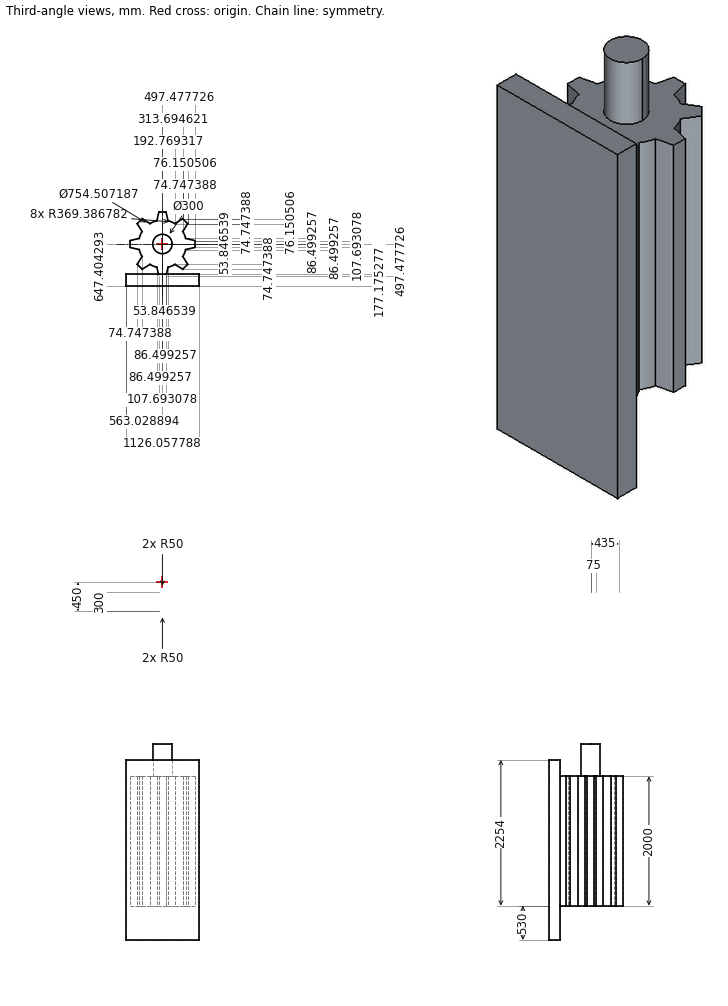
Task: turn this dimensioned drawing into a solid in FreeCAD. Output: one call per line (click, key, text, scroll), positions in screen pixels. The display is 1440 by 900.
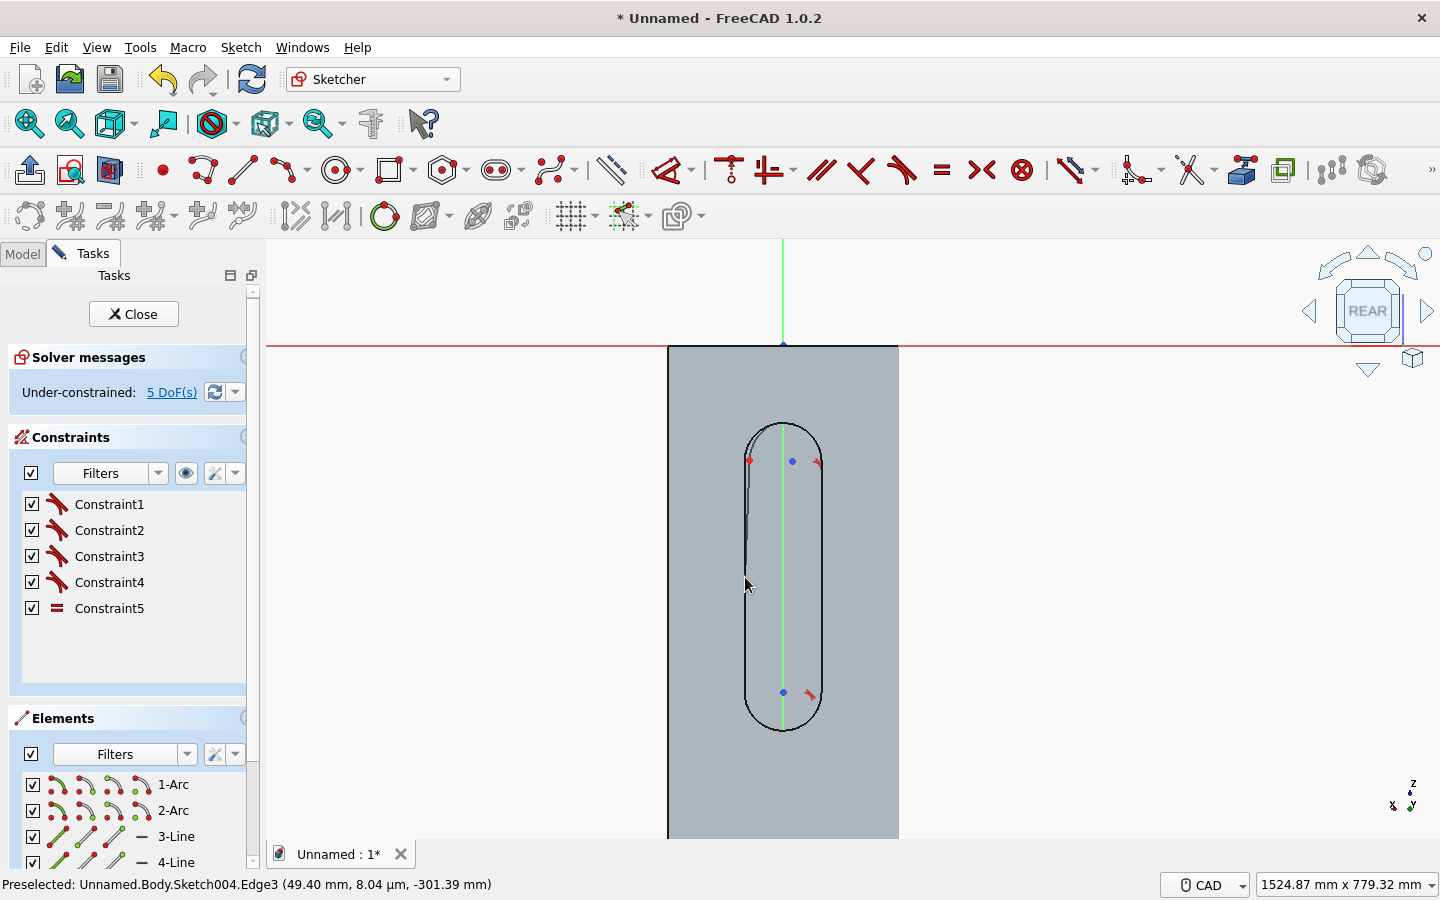
click(743, 622)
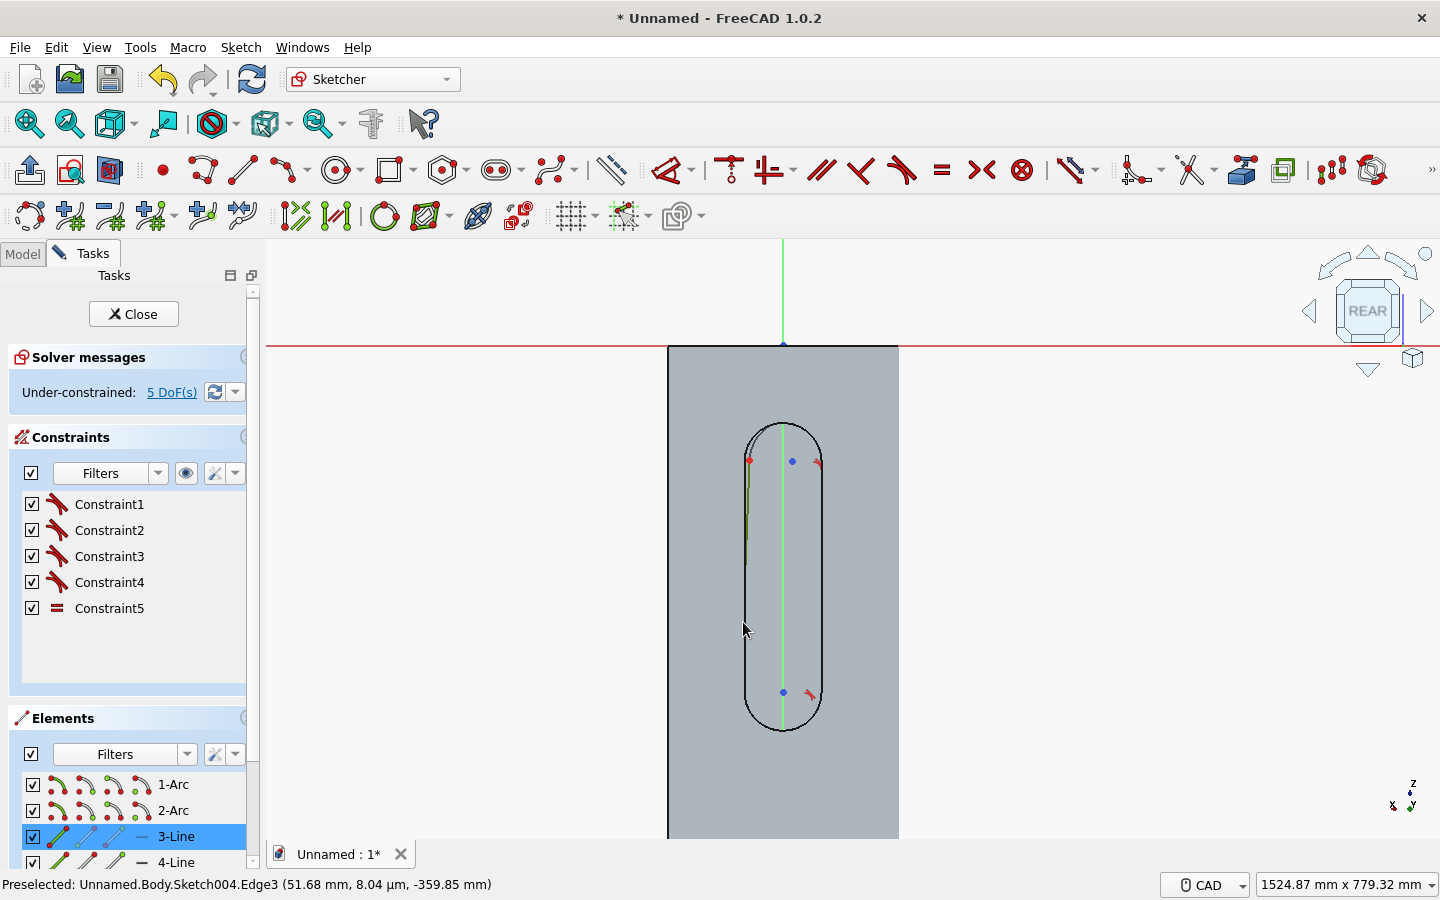
key(v)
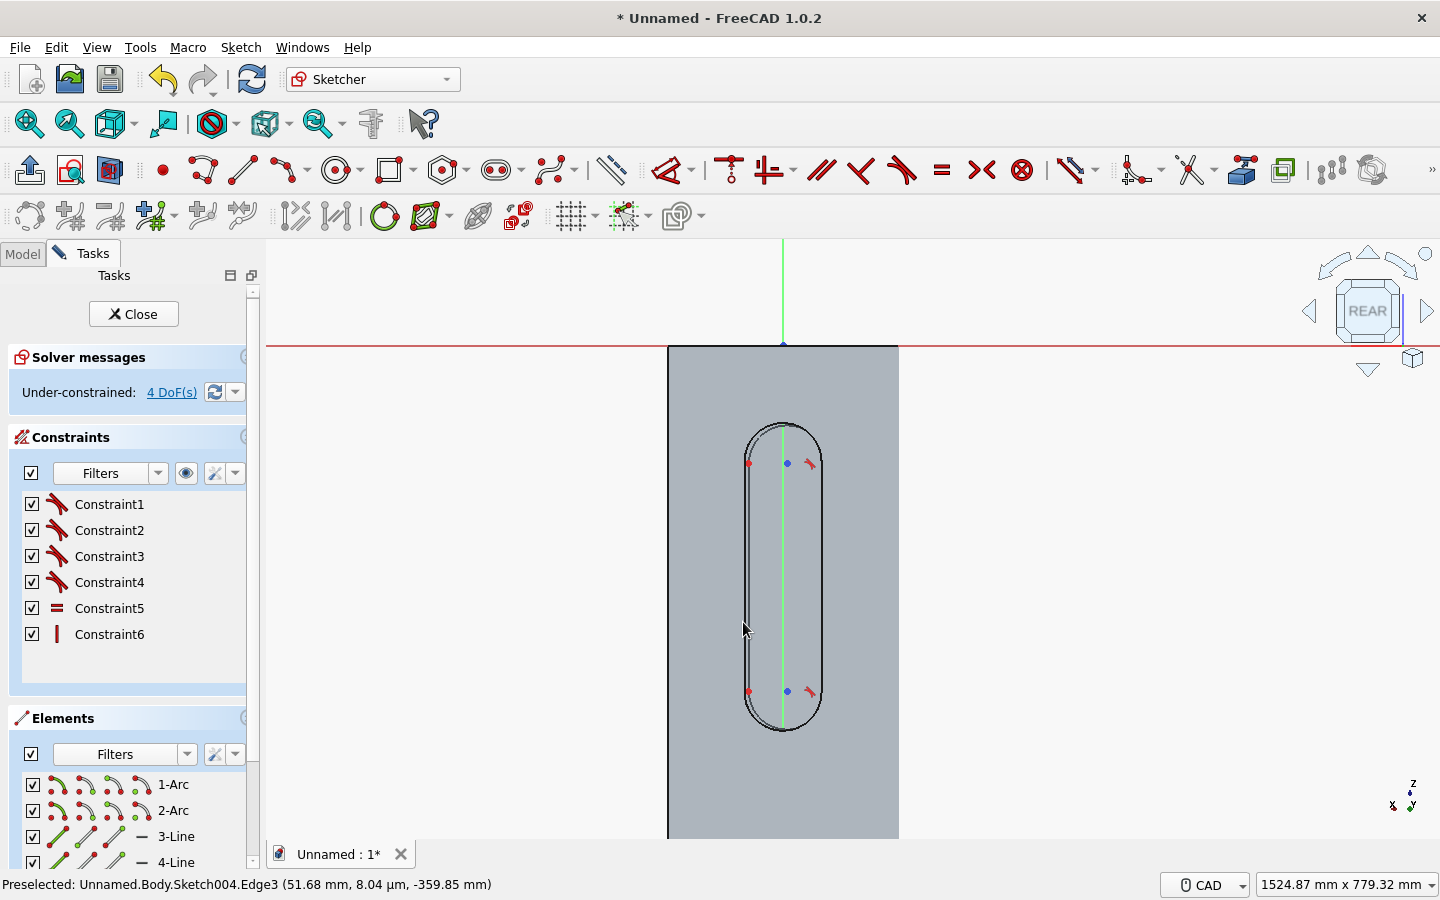
click(787, 691)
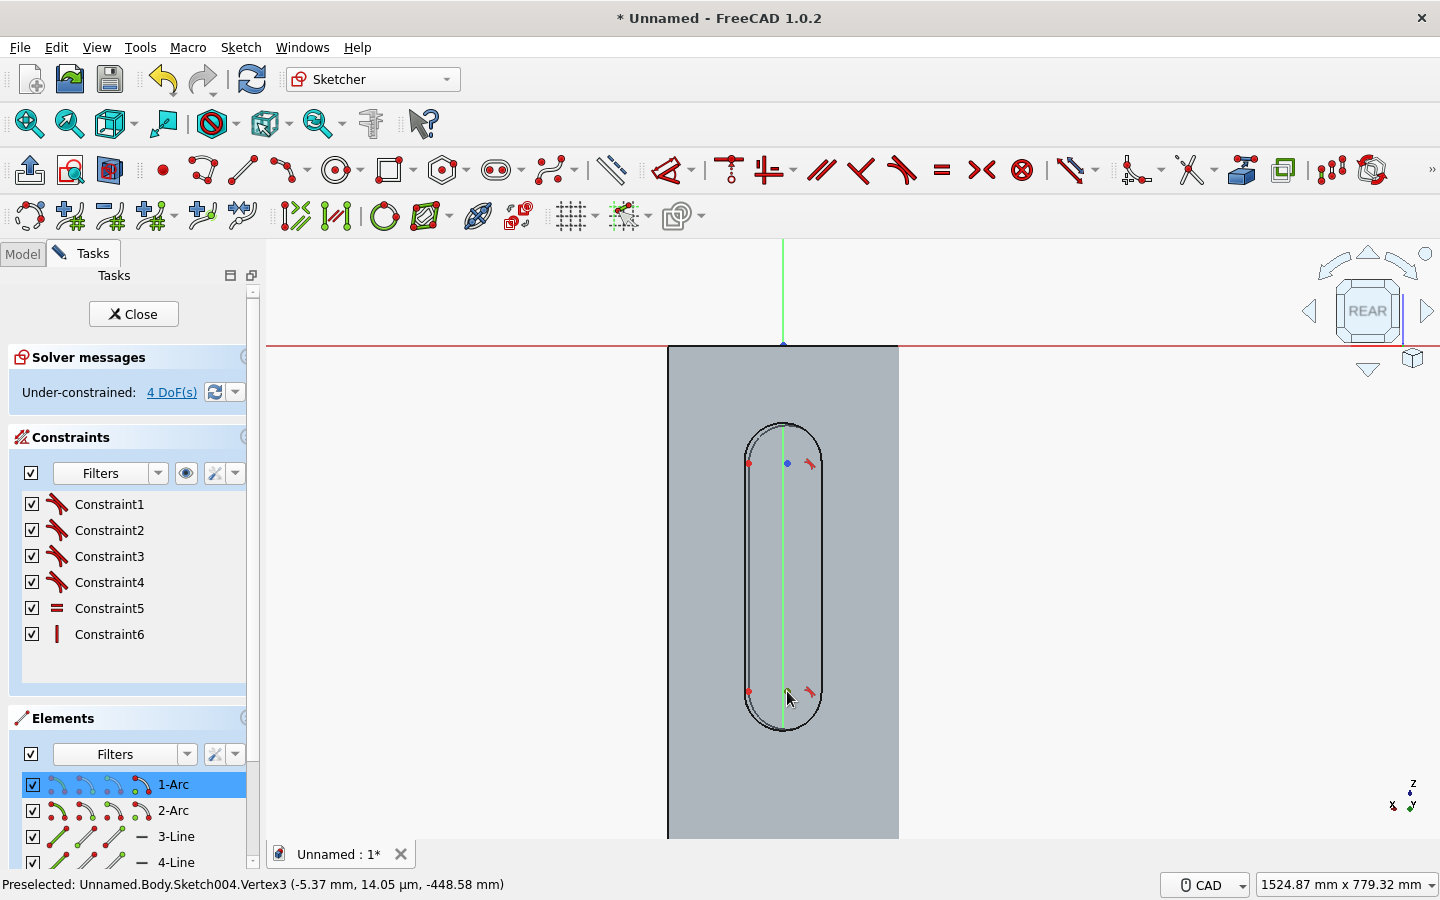
click(783, 772)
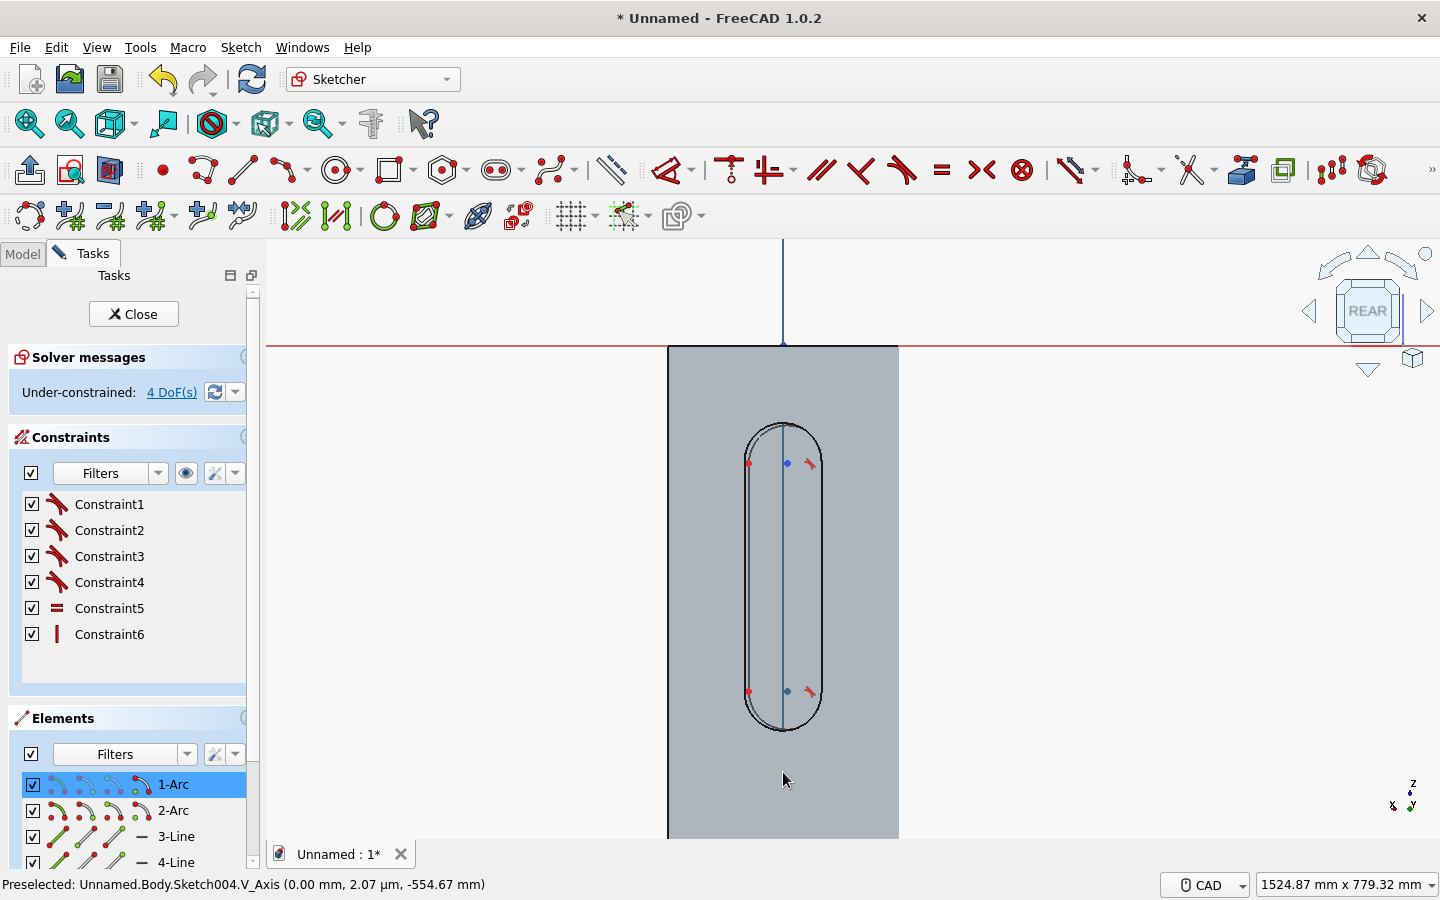
click(730, 170)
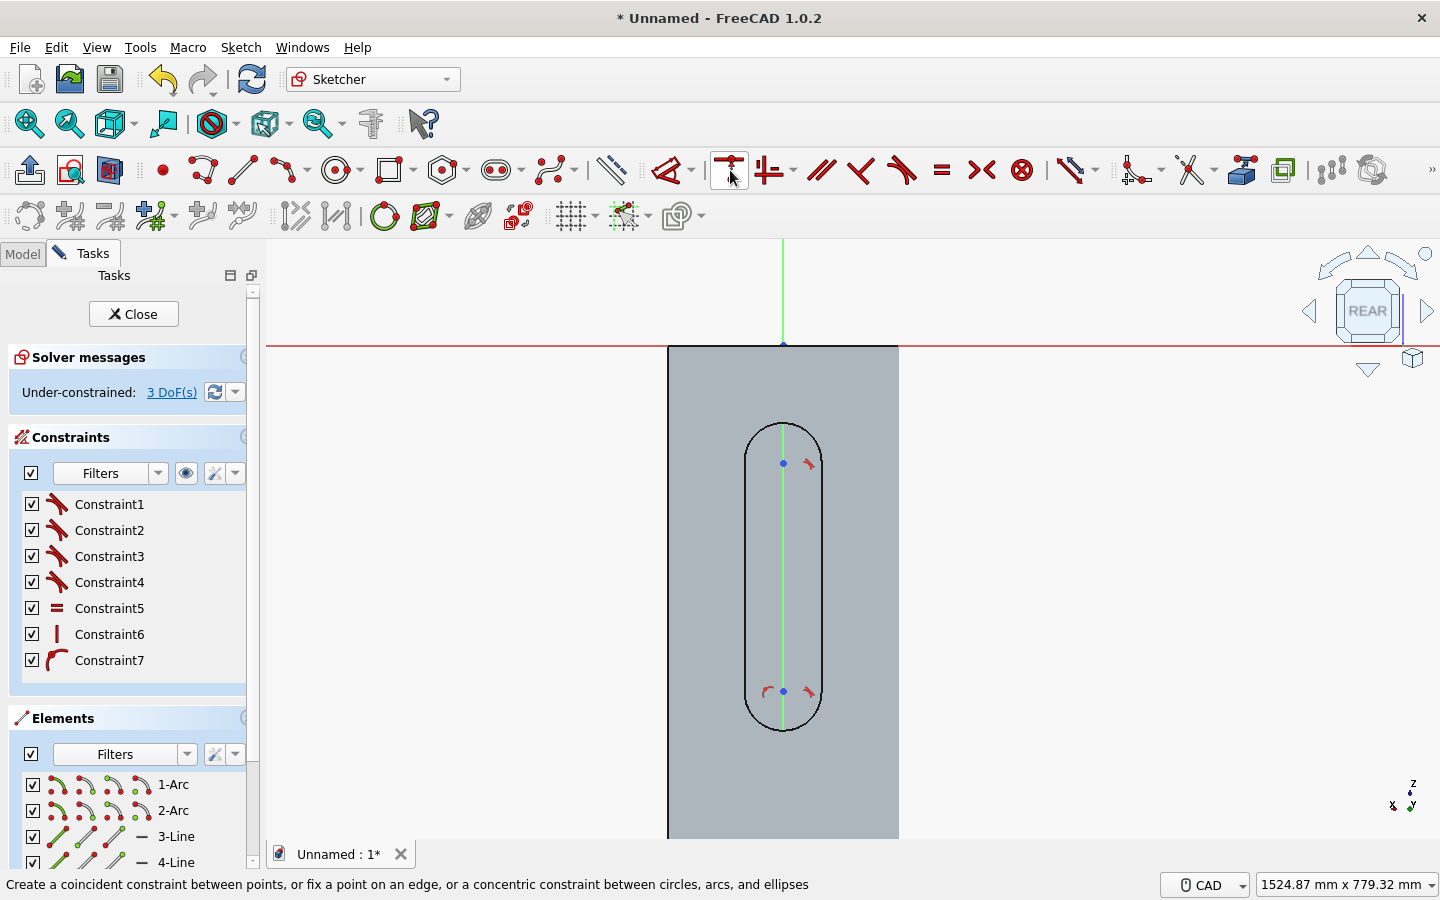
click(666, 170)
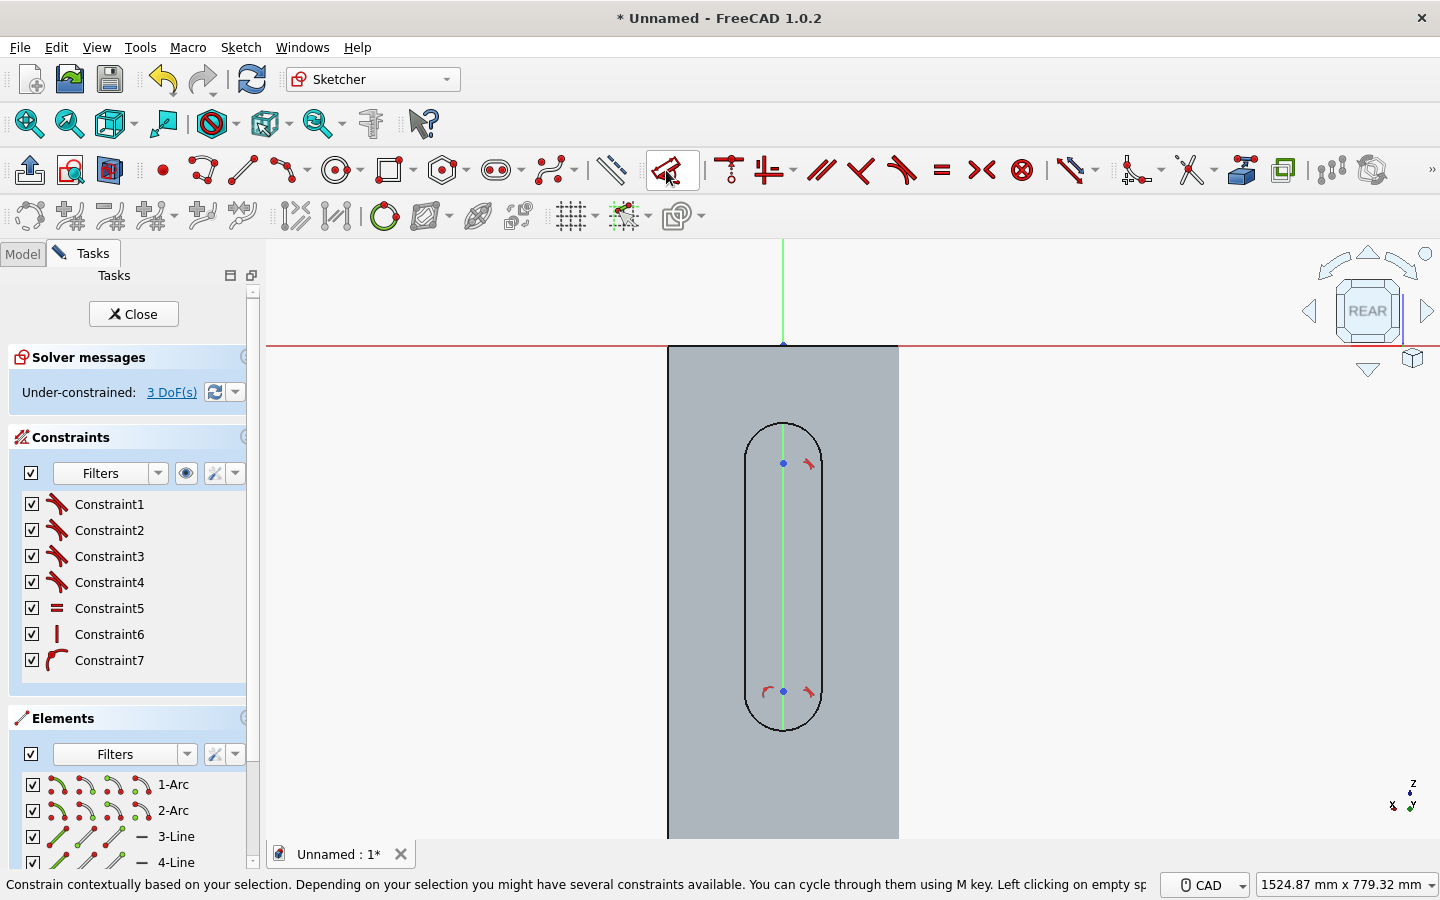
click(759, 725)
click(740, 751)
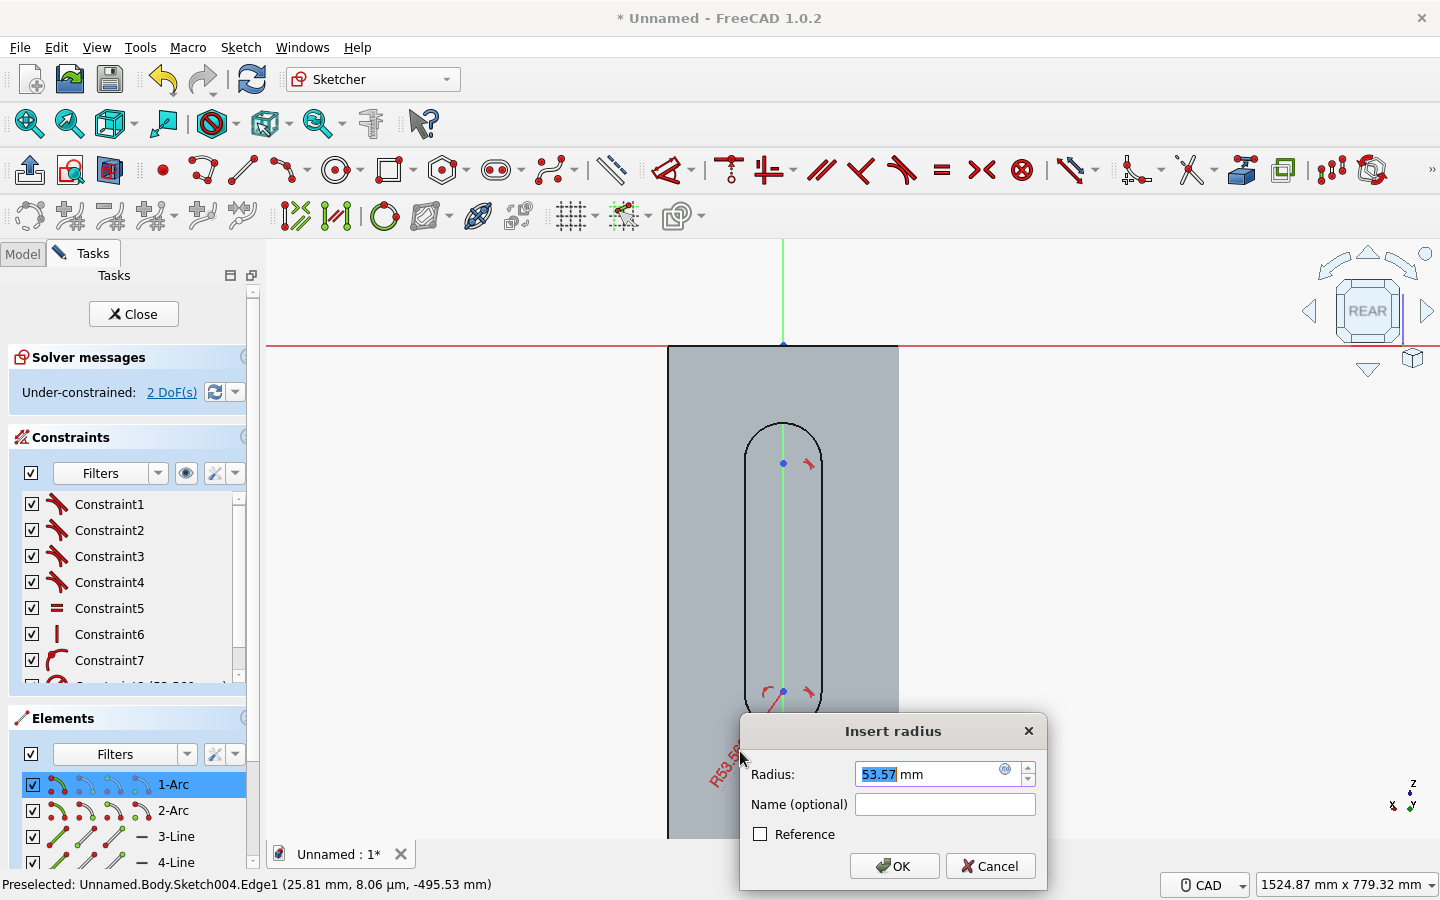
text(50)
key(Return)